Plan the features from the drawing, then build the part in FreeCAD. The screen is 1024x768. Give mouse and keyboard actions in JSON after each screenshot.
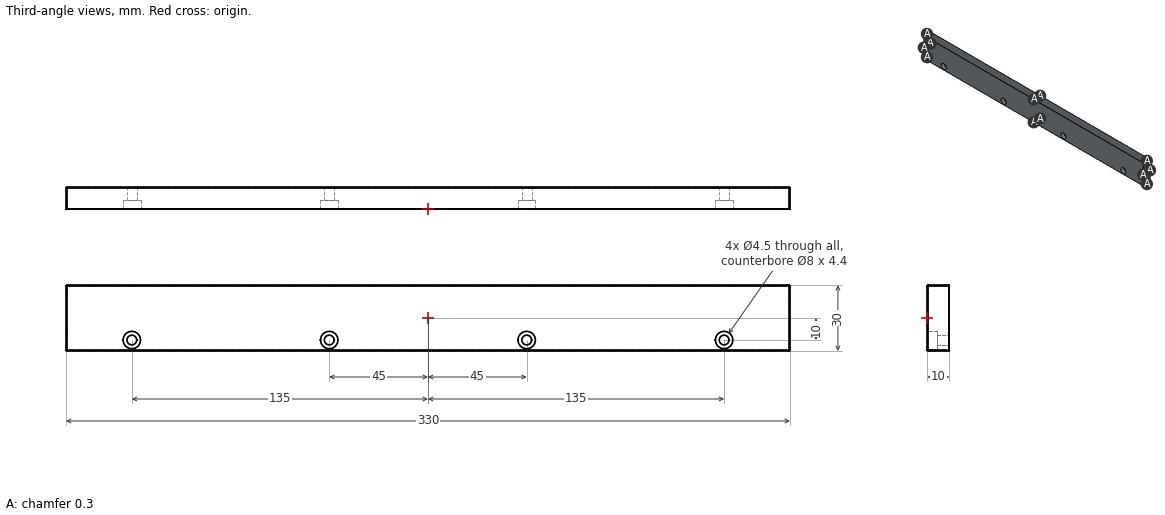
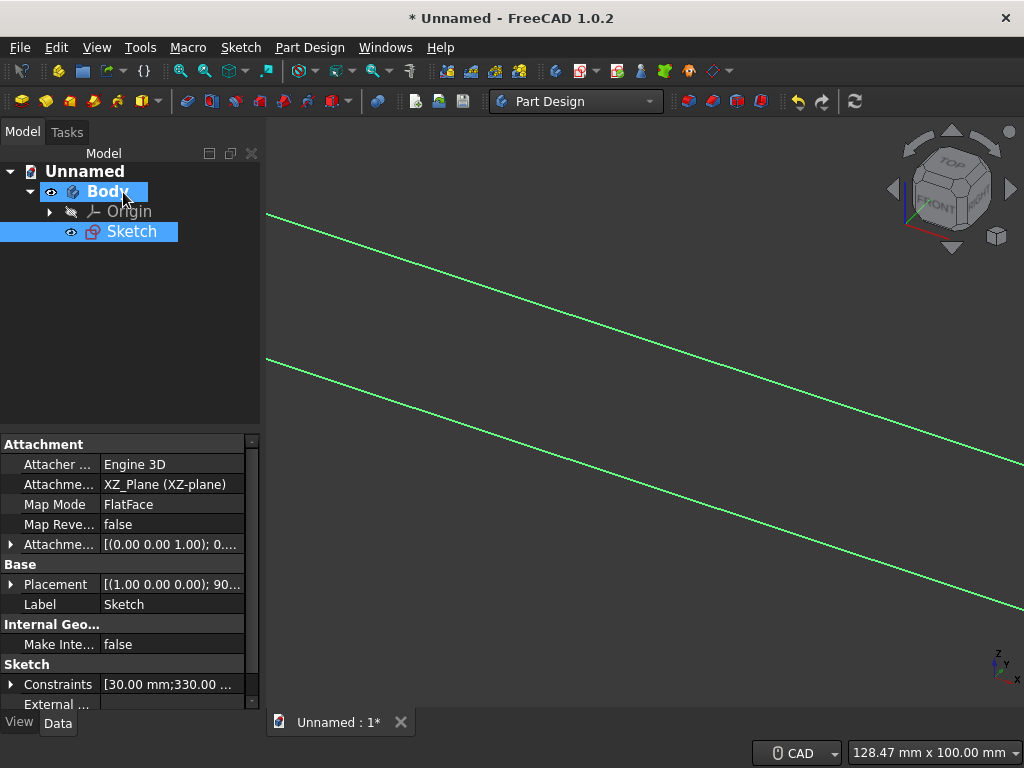
{"action": "left_click", "coordinate": [22, 102]}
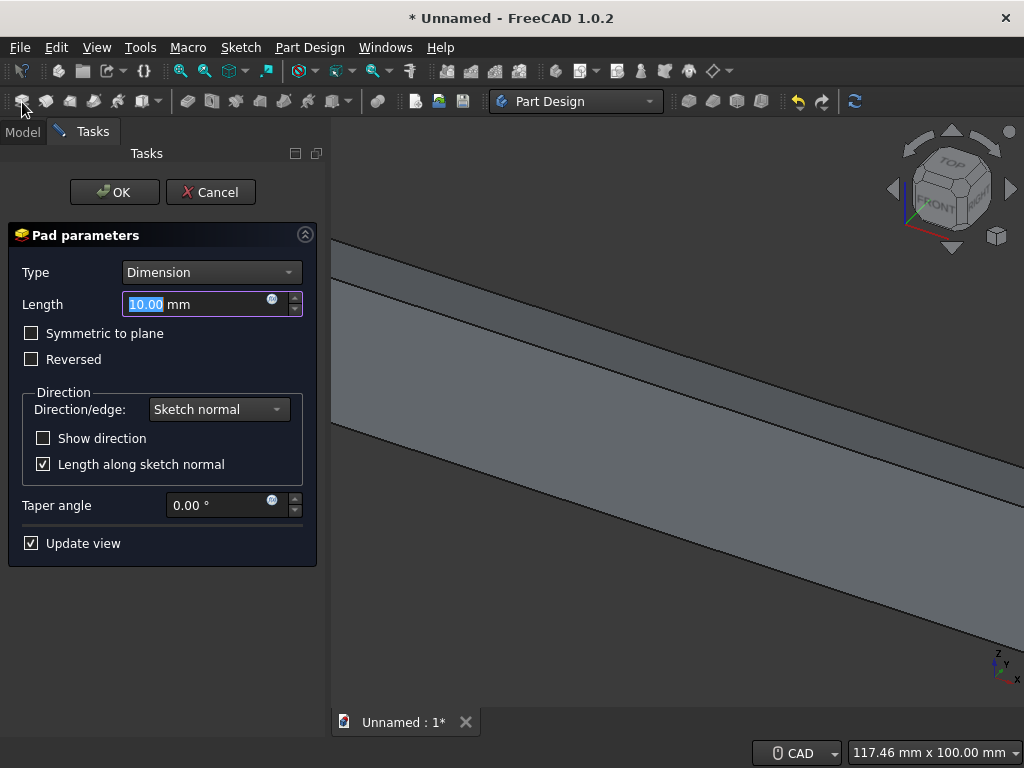
{"action": "type", "text": "10"}
{"action": "key", "text": "Tab"}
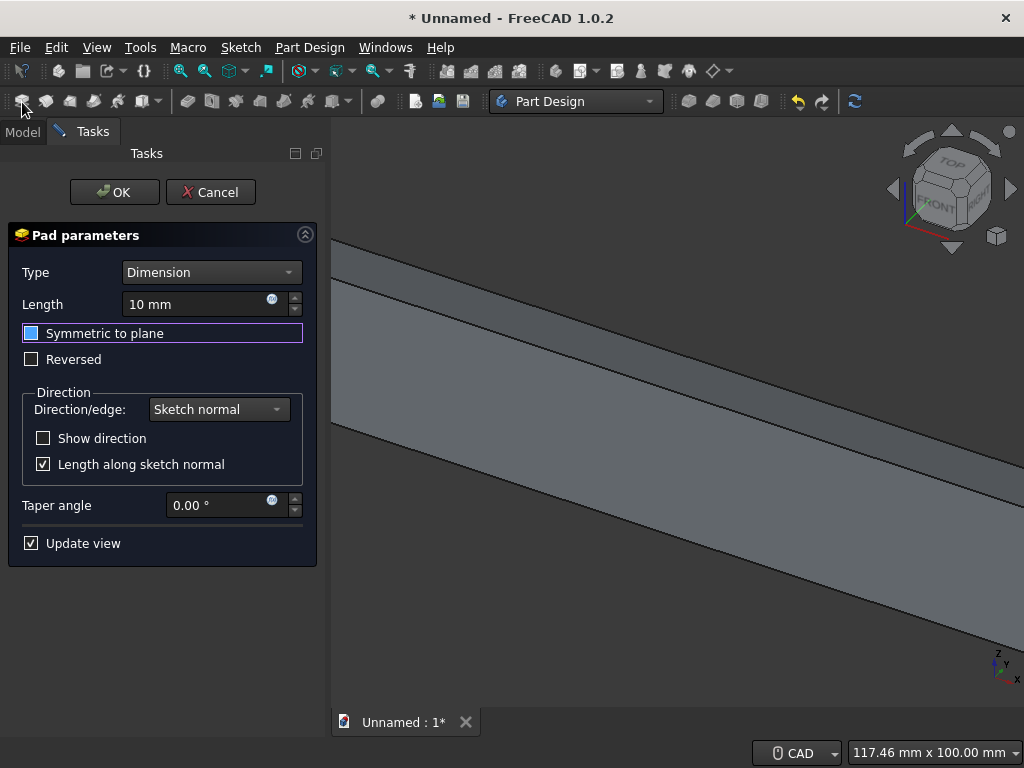
{"action": "left_click", "coordinate": [30, 359]}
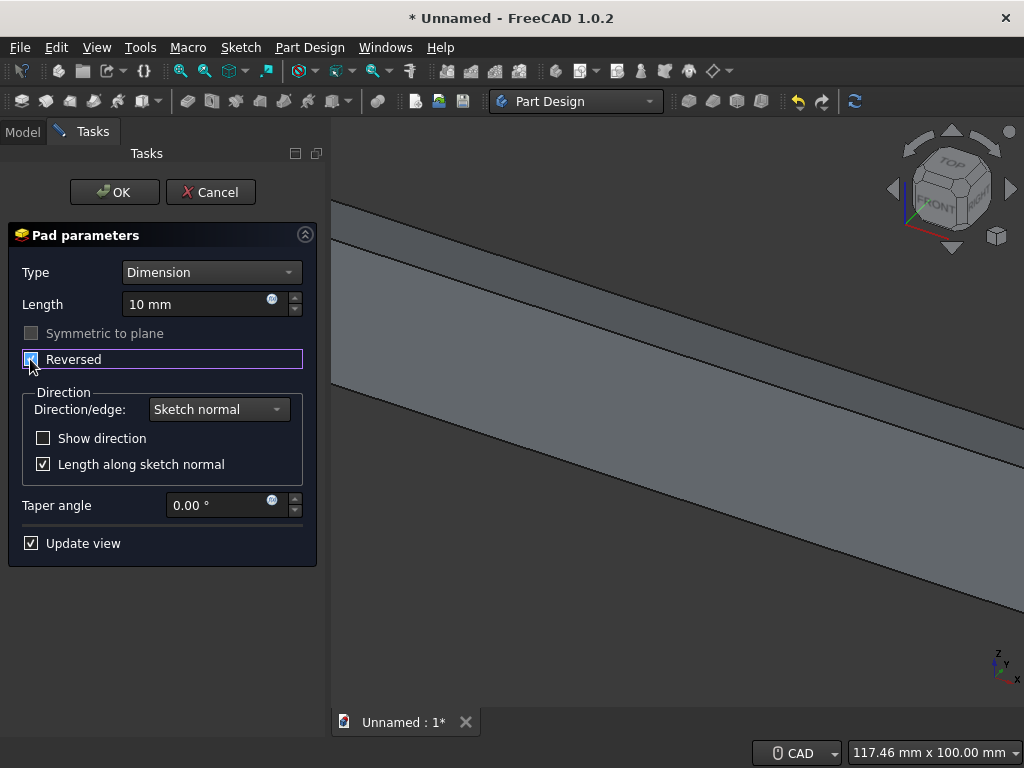
{"action": "left_click", "coordinate": [115, 192]}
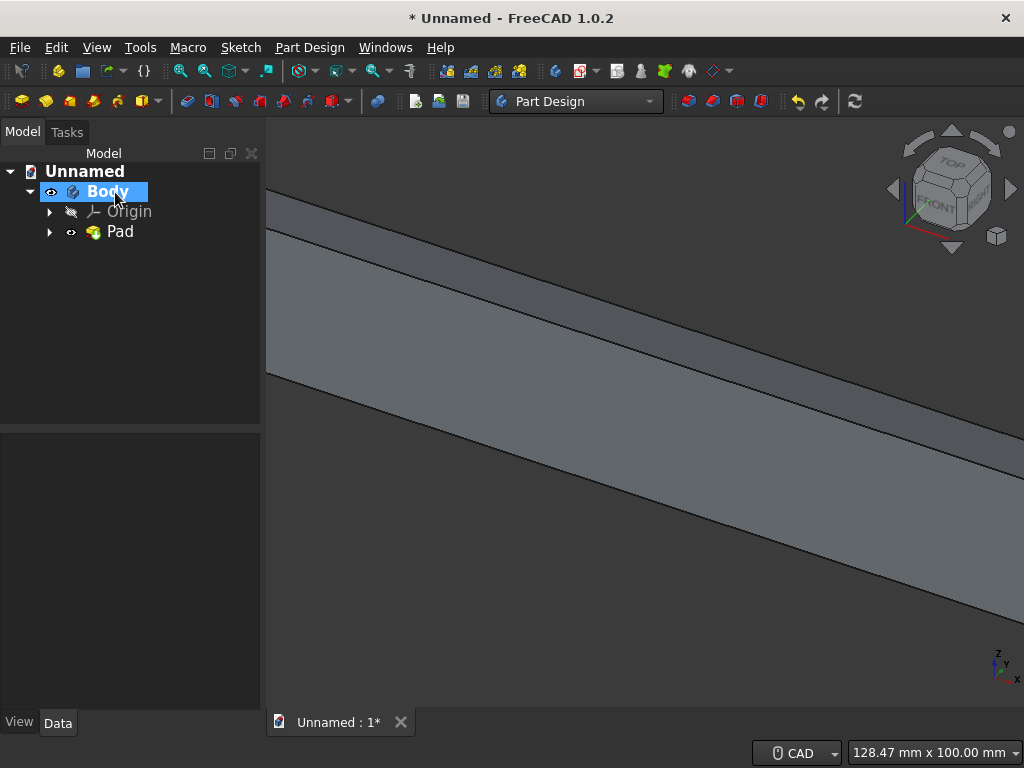
{"action": "key", "text": "v f"}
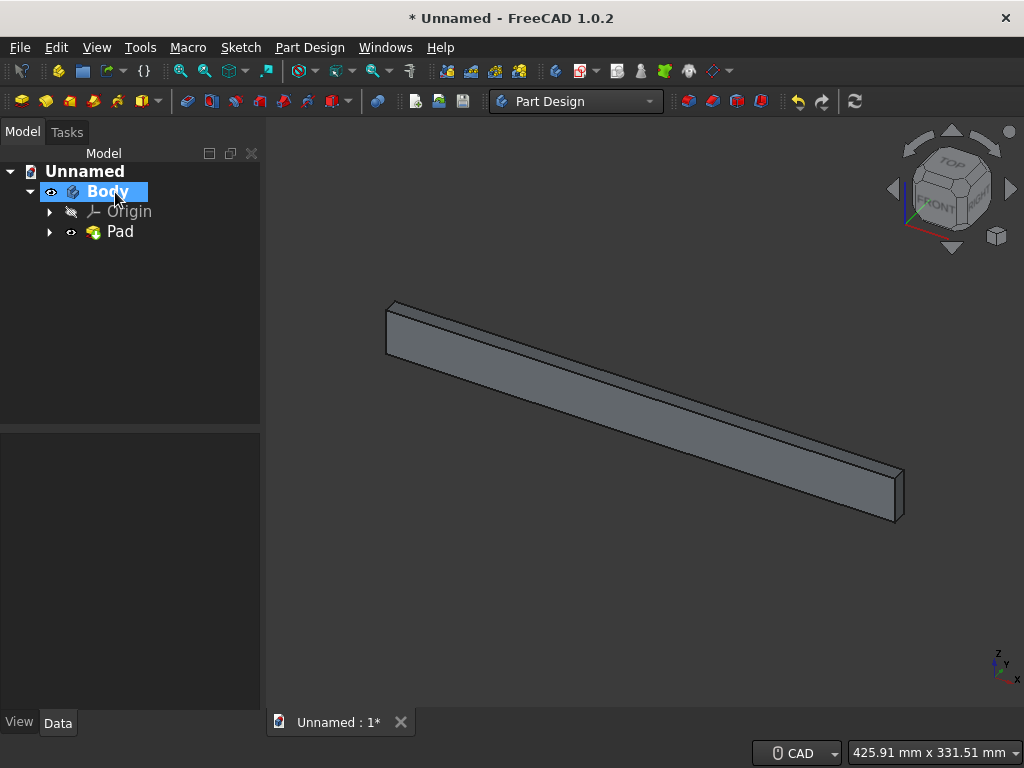
{"action": "left_click", "coordinate": [859, 488]}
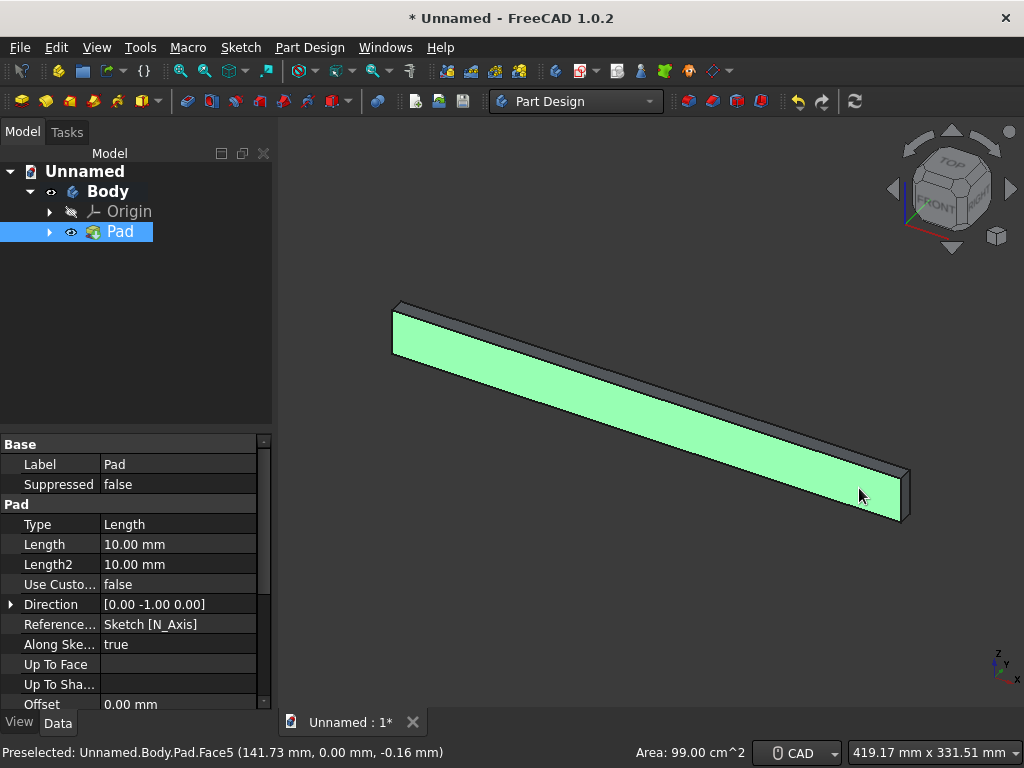
{"action": "left_click", "coordinate": [580, 72]}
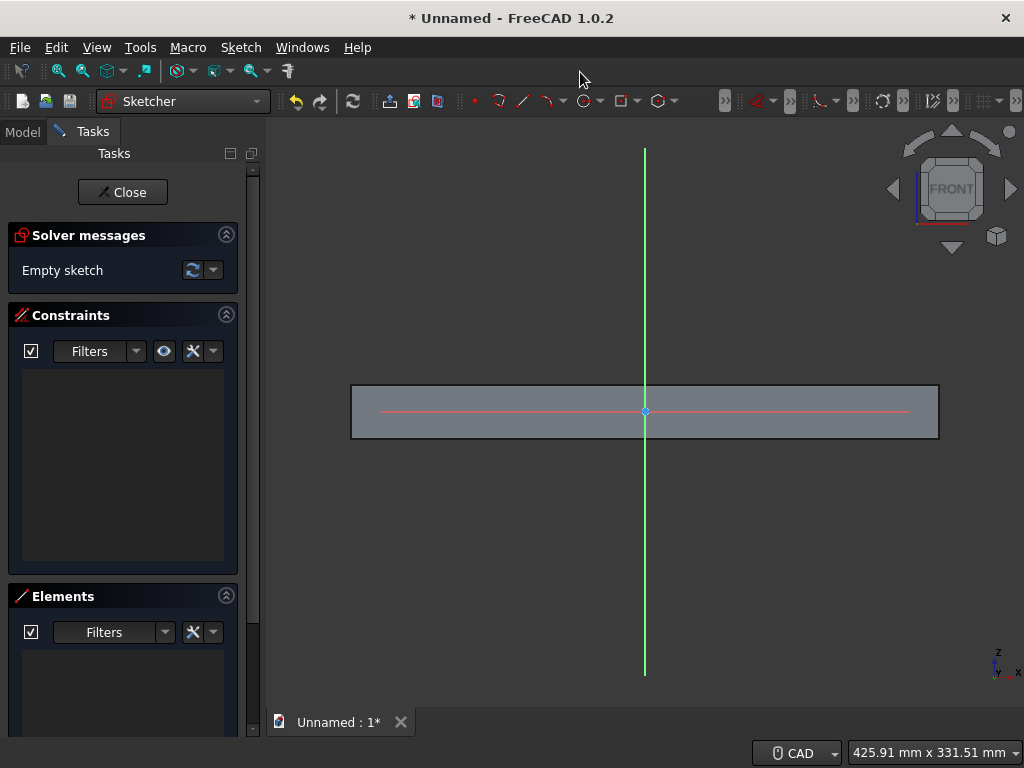
{"action": "scroll", "coordinate": [294, 363], "scroll_direction": "down", "scroll_amount": 1}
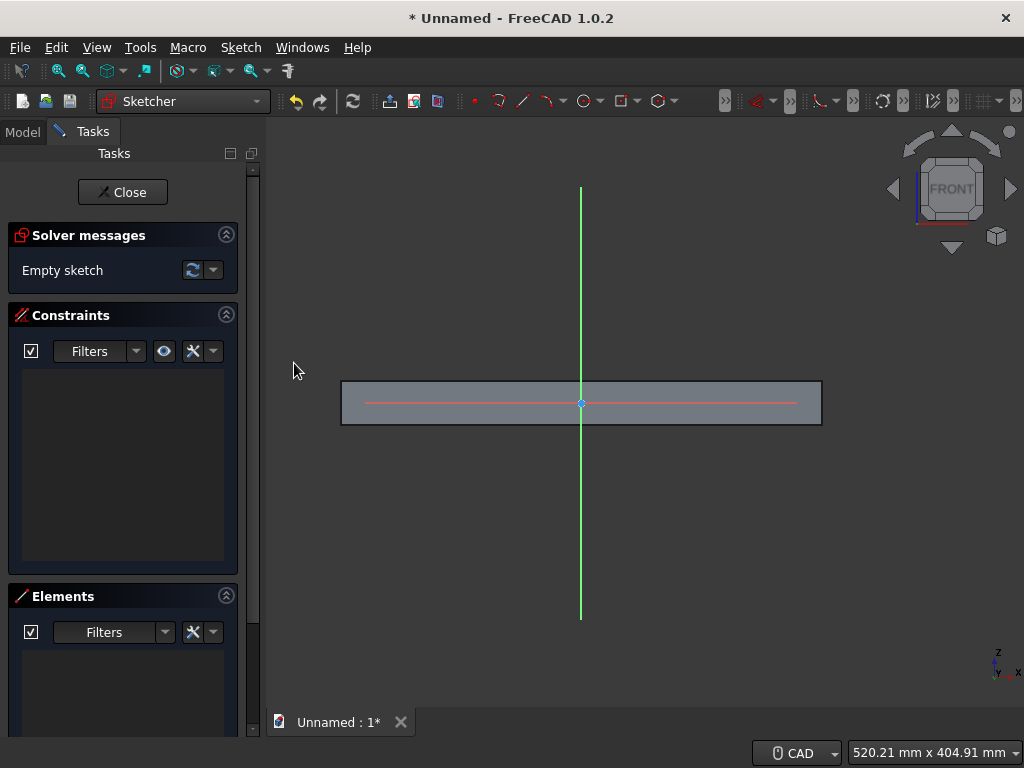
{"action": "key", "text": "g c"}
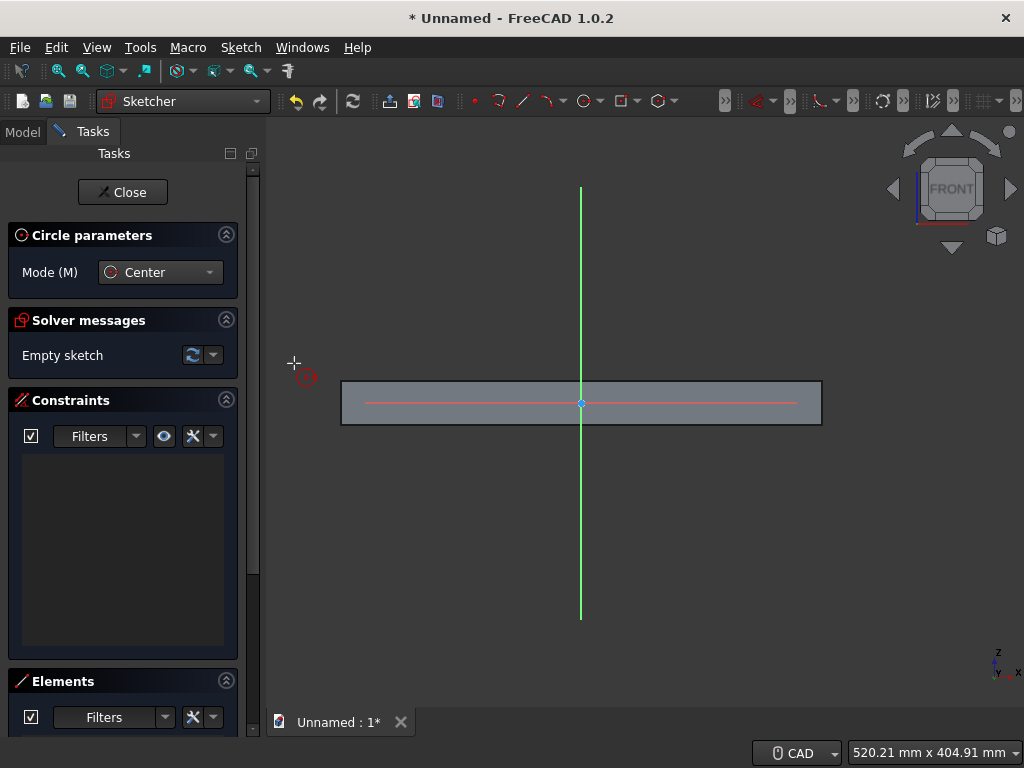
{"action": "scroll", "coordinate": [778, 418], "scroll_direction": "up", "scroll_amount": 10}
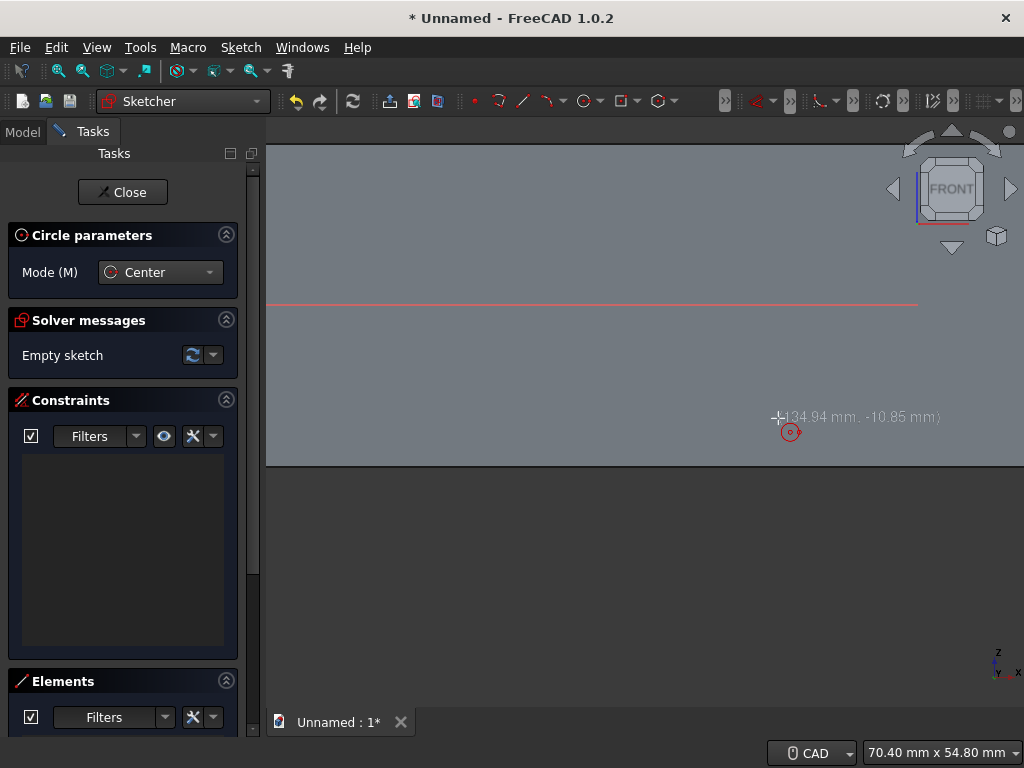
{"action": "scroll", "coordinate": [773, 418], "scroll_direction": "down", "scroll_amount": 10}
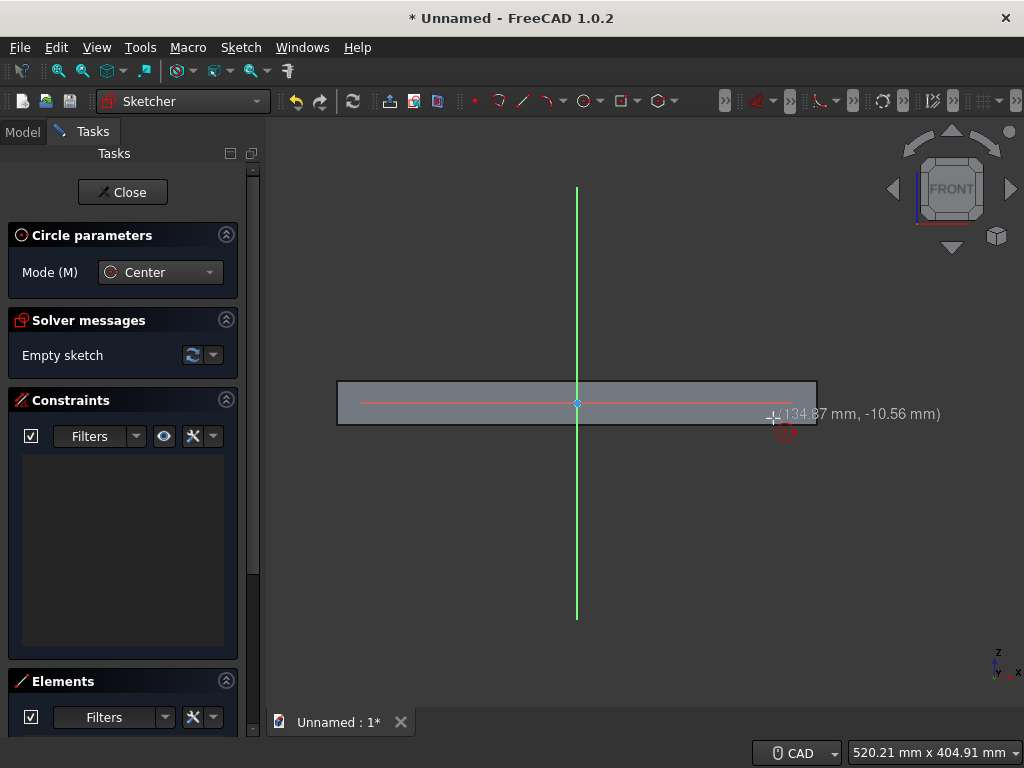
{"action": "left_click", "coordinate": [774, 418]}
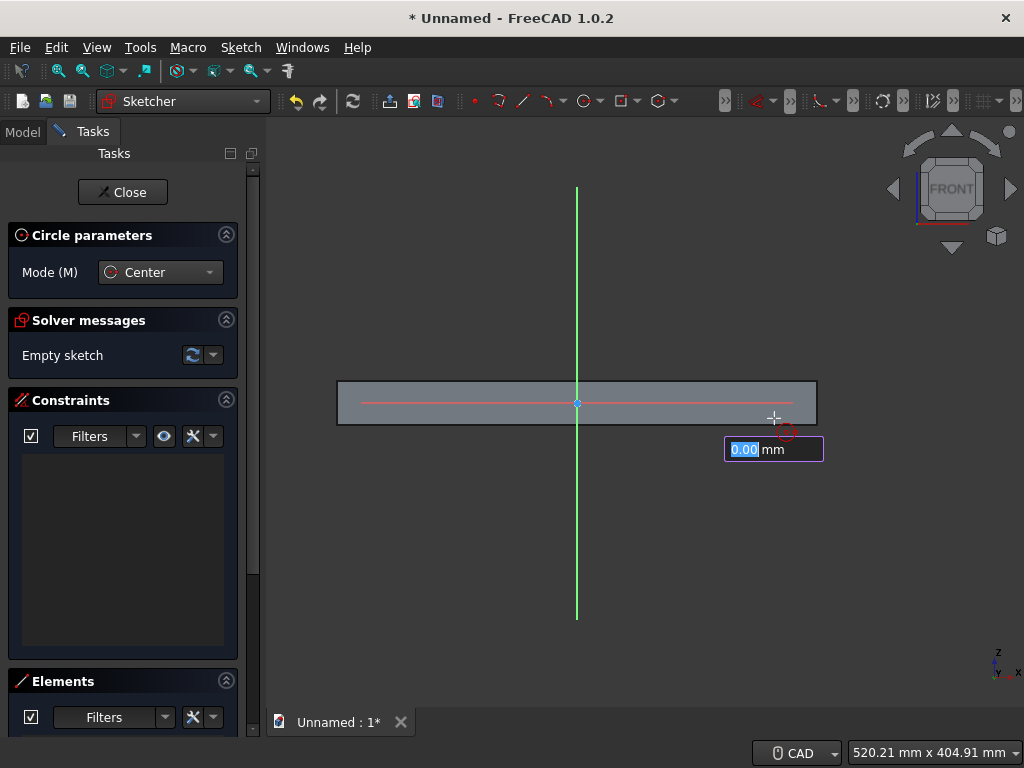
{"action": "scroll", "coordinate": [776, 420], "scroll_direction": "up", "scroll_amount": 8}